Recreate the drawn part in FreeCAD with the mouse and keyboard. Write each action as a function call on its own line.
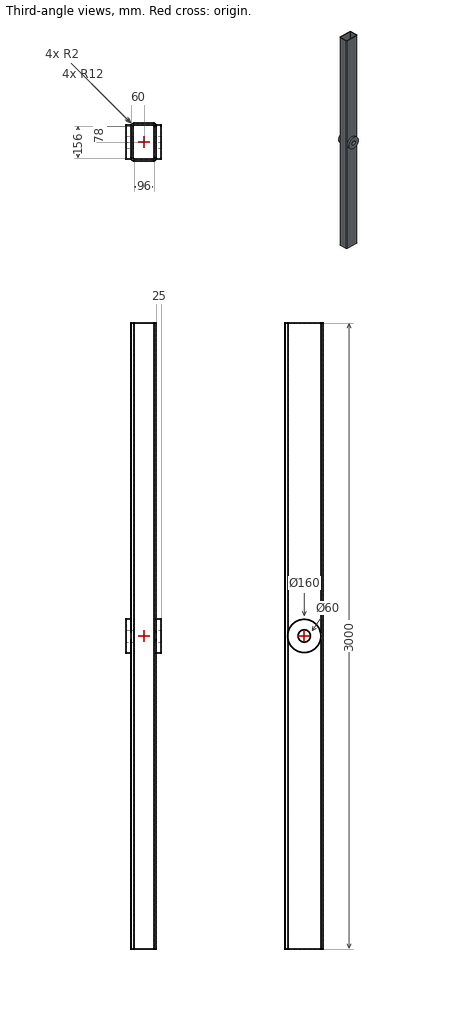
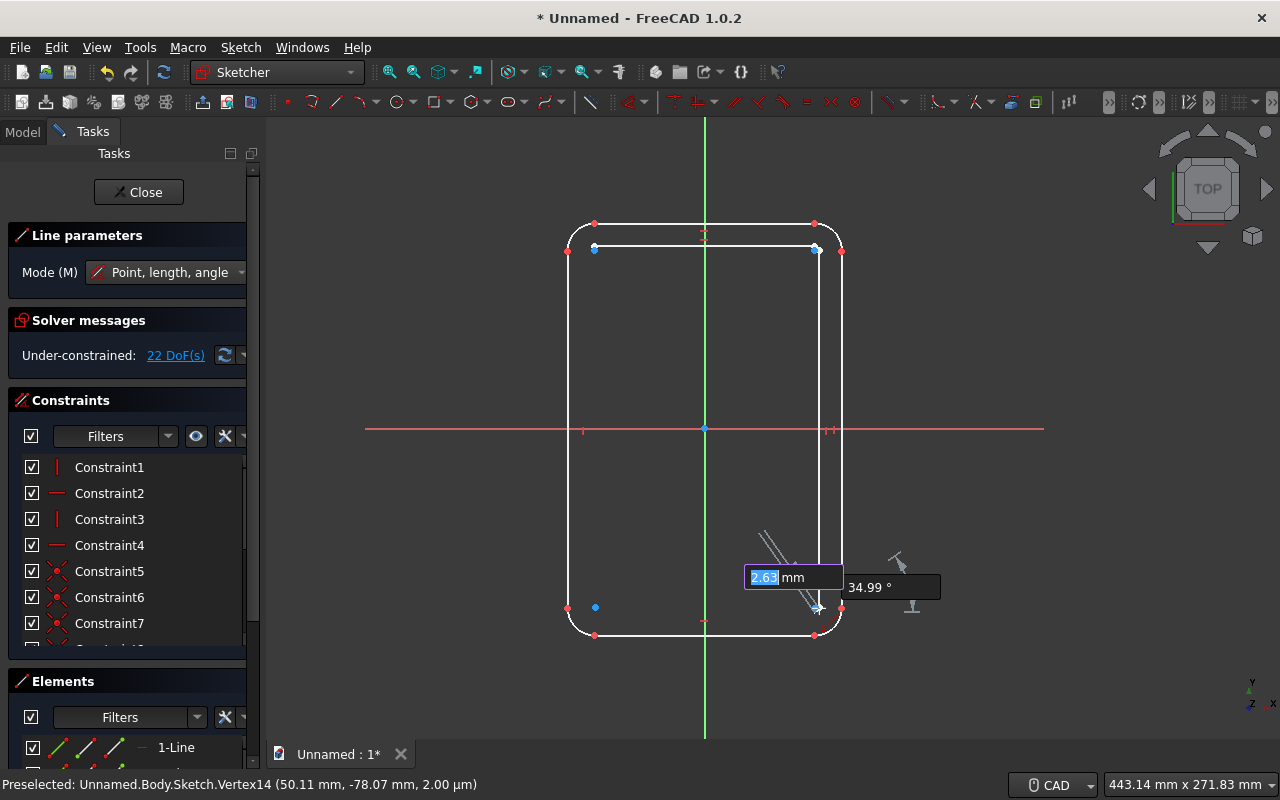
scroll(595, 612, up, 7)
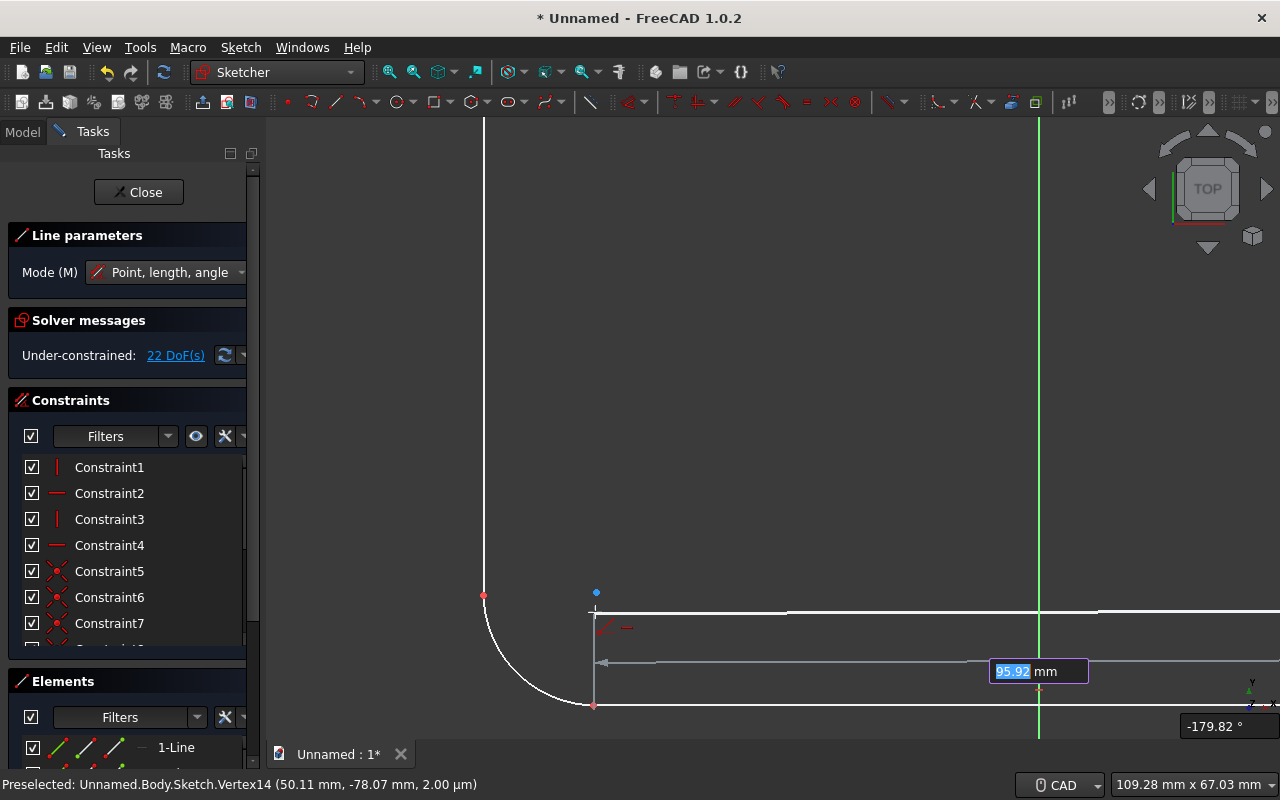
click(594, 610)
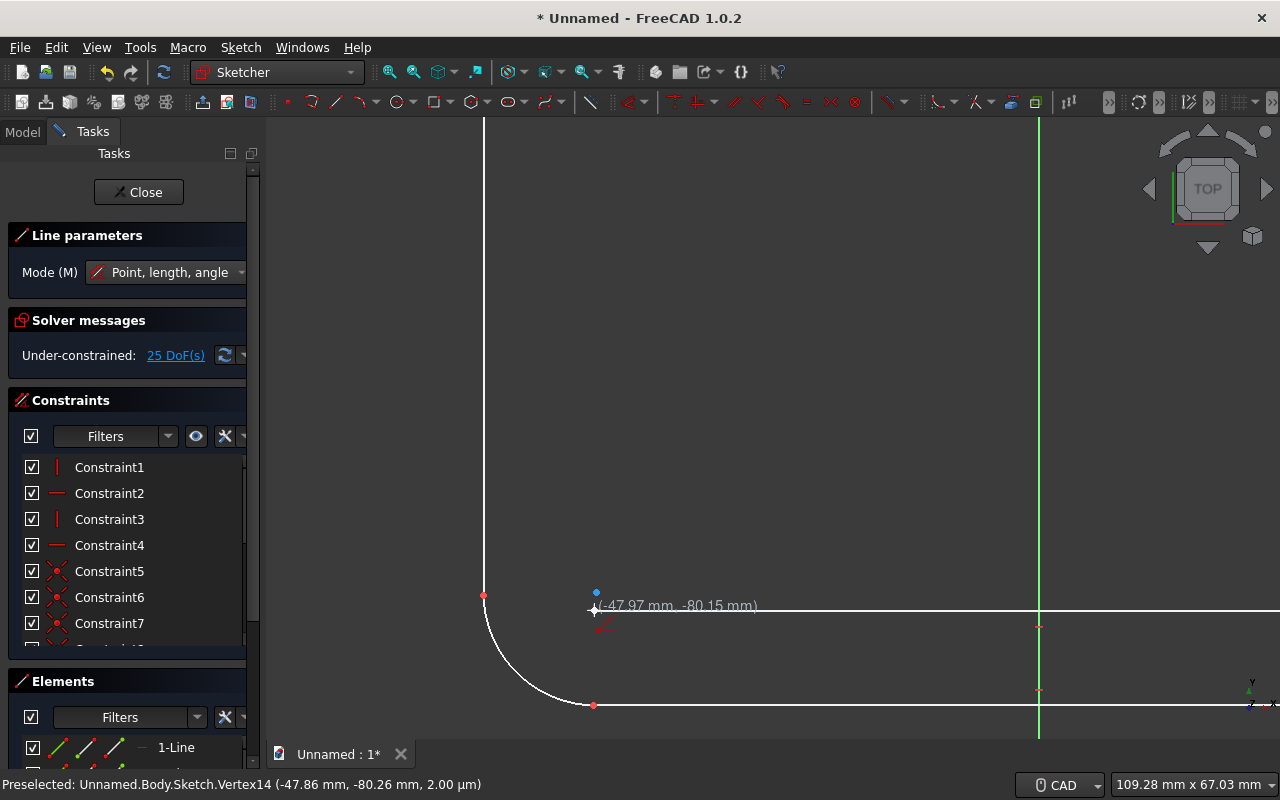
click(575, 591)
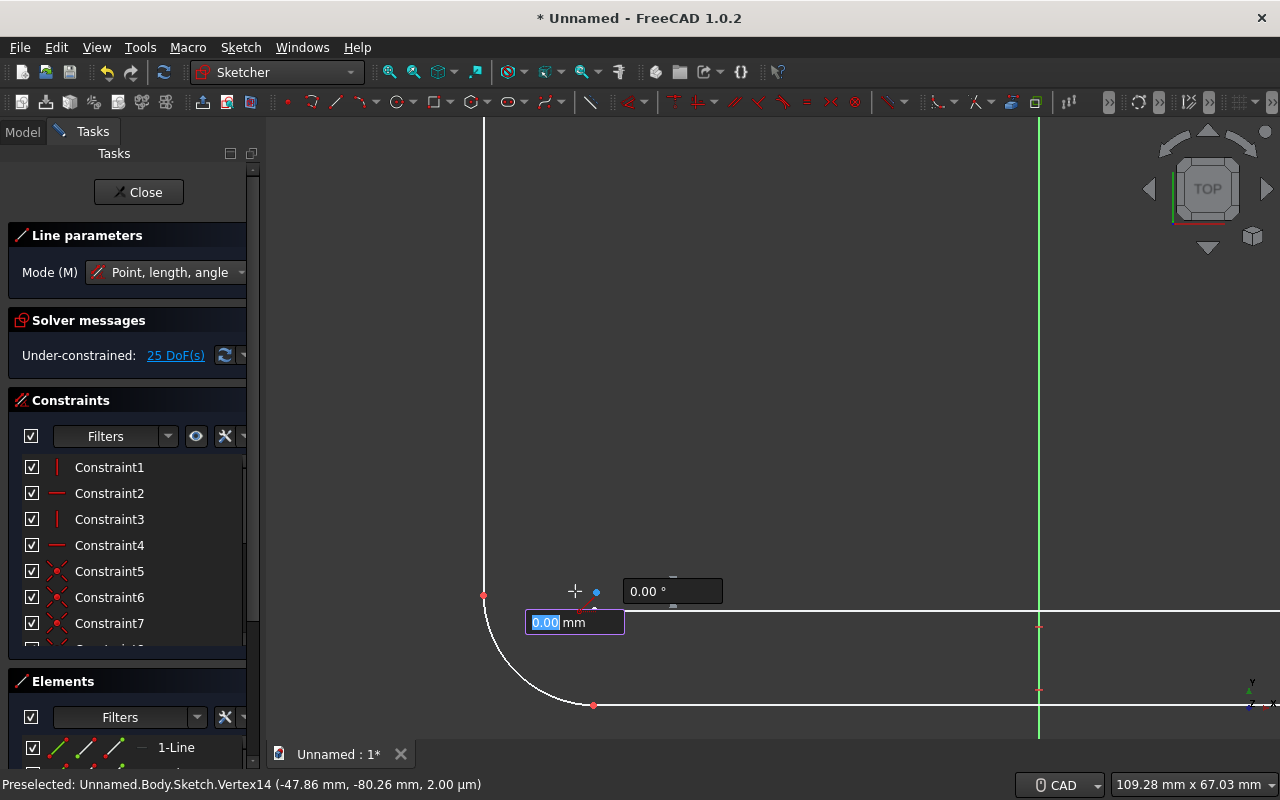
scroll(595, 612, down, 7)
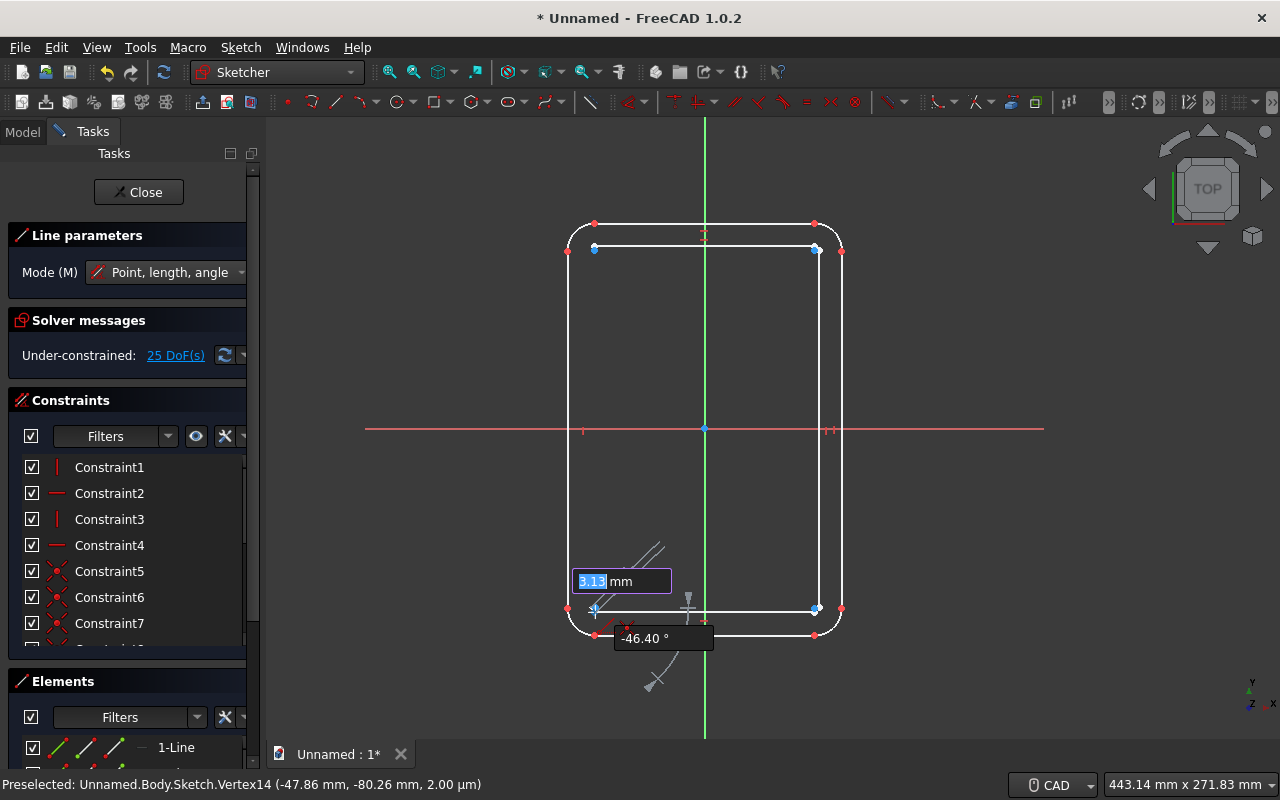
scroll(590, 250, up, 7)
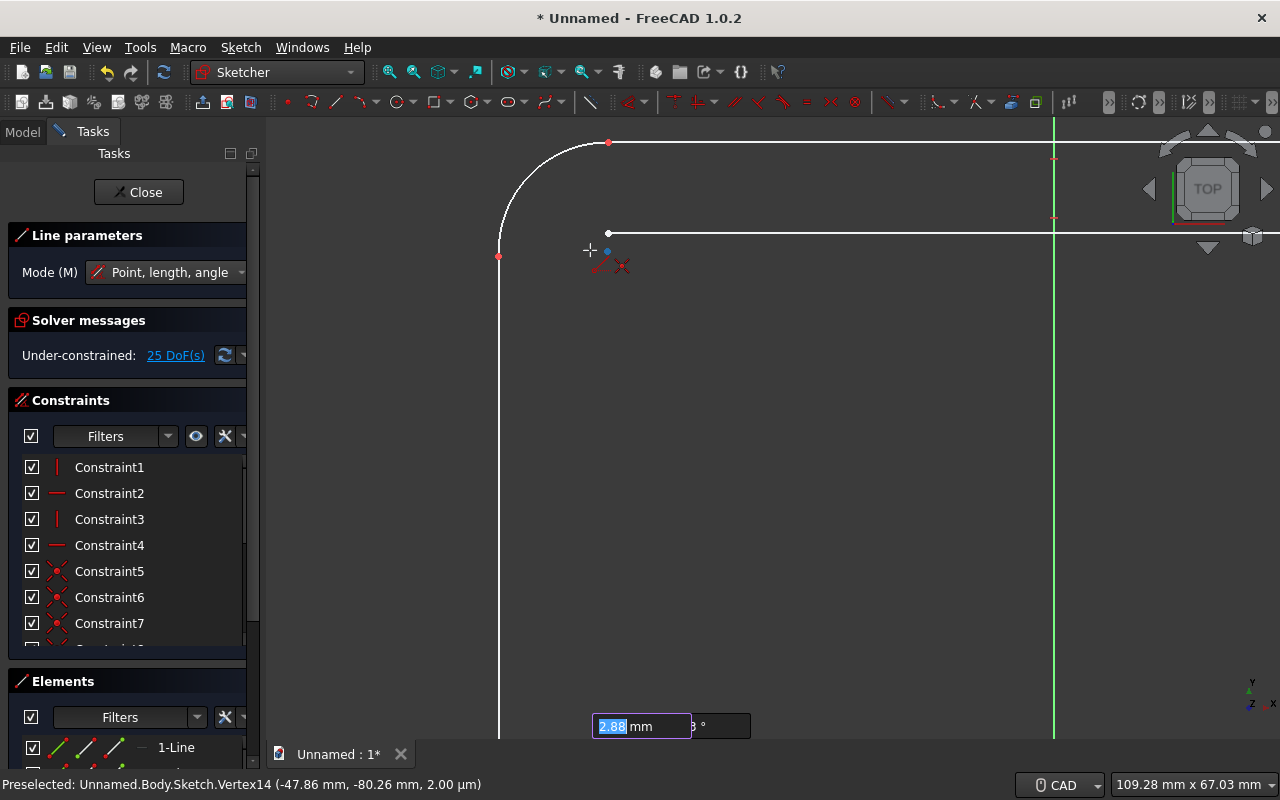
click(590, 251)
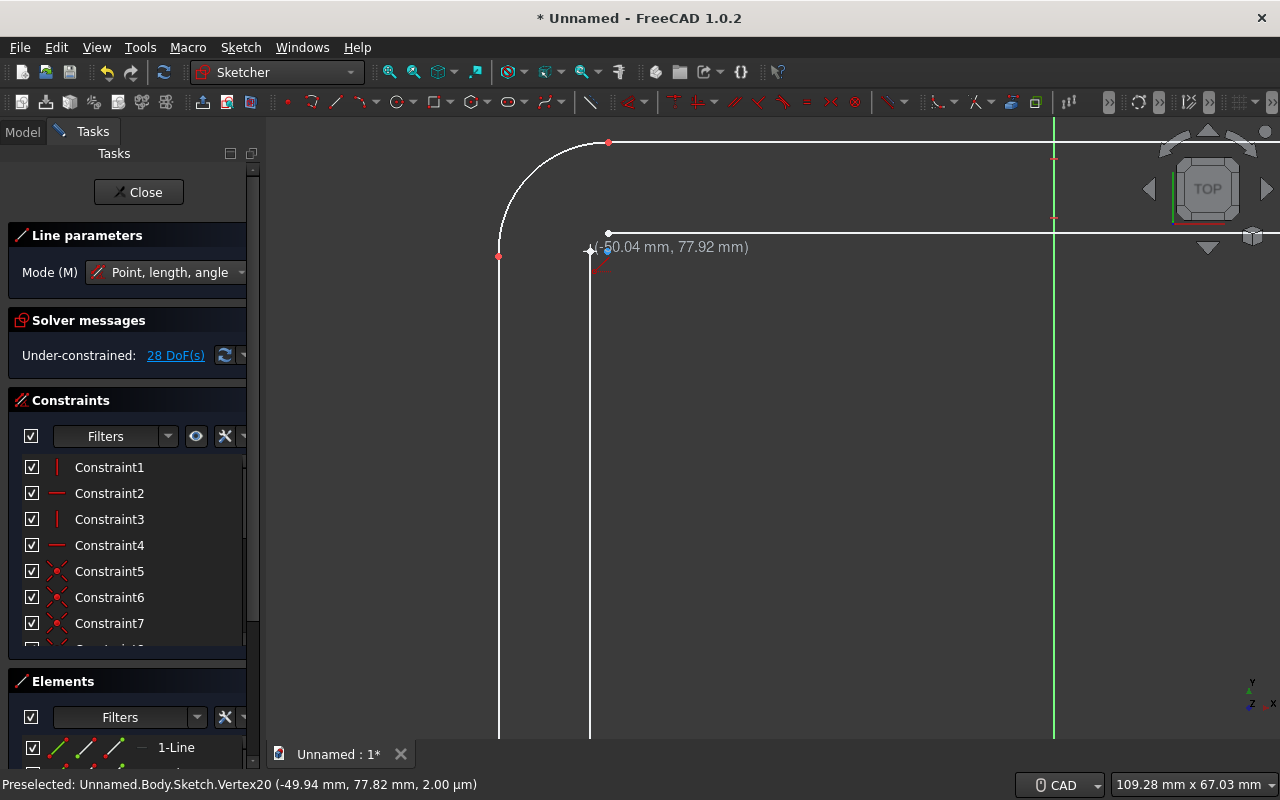
click(360, 102)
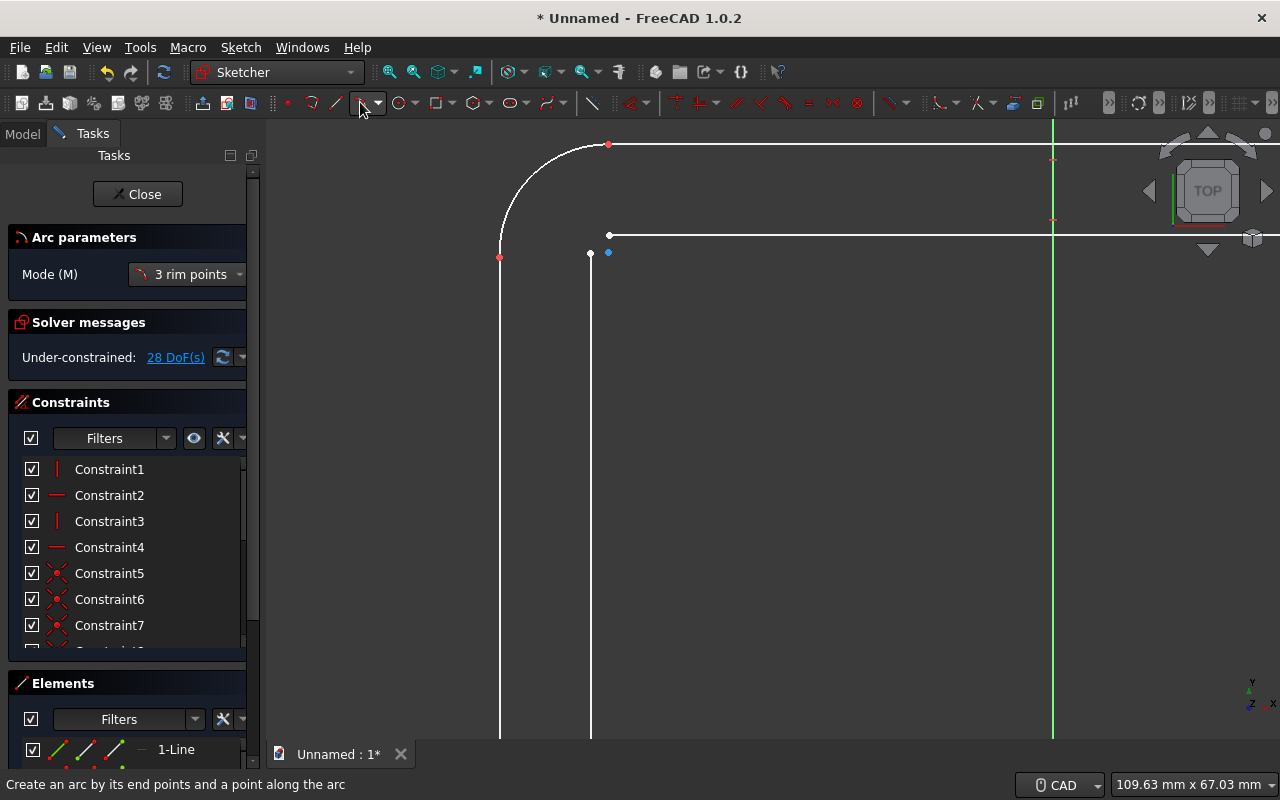
scroll(590, 251, down, 7)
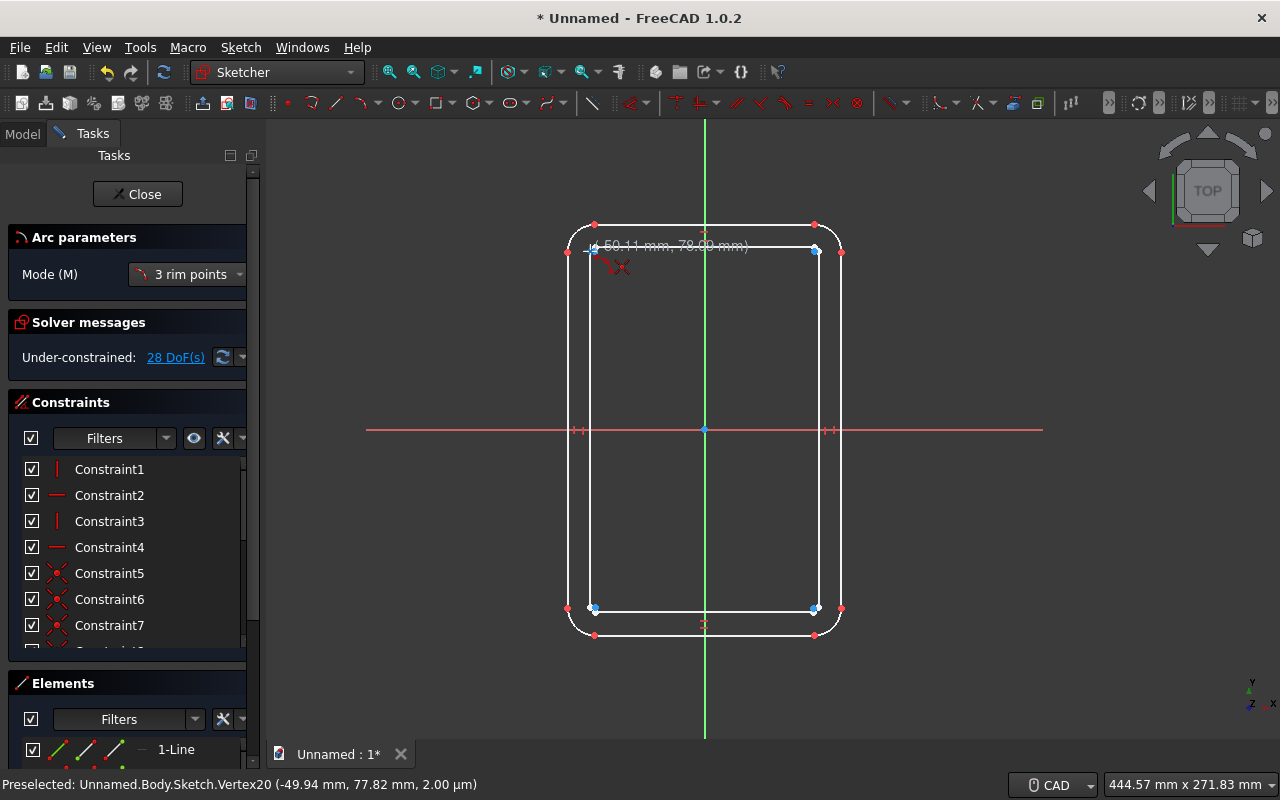
scroll(814, 247, up, 7)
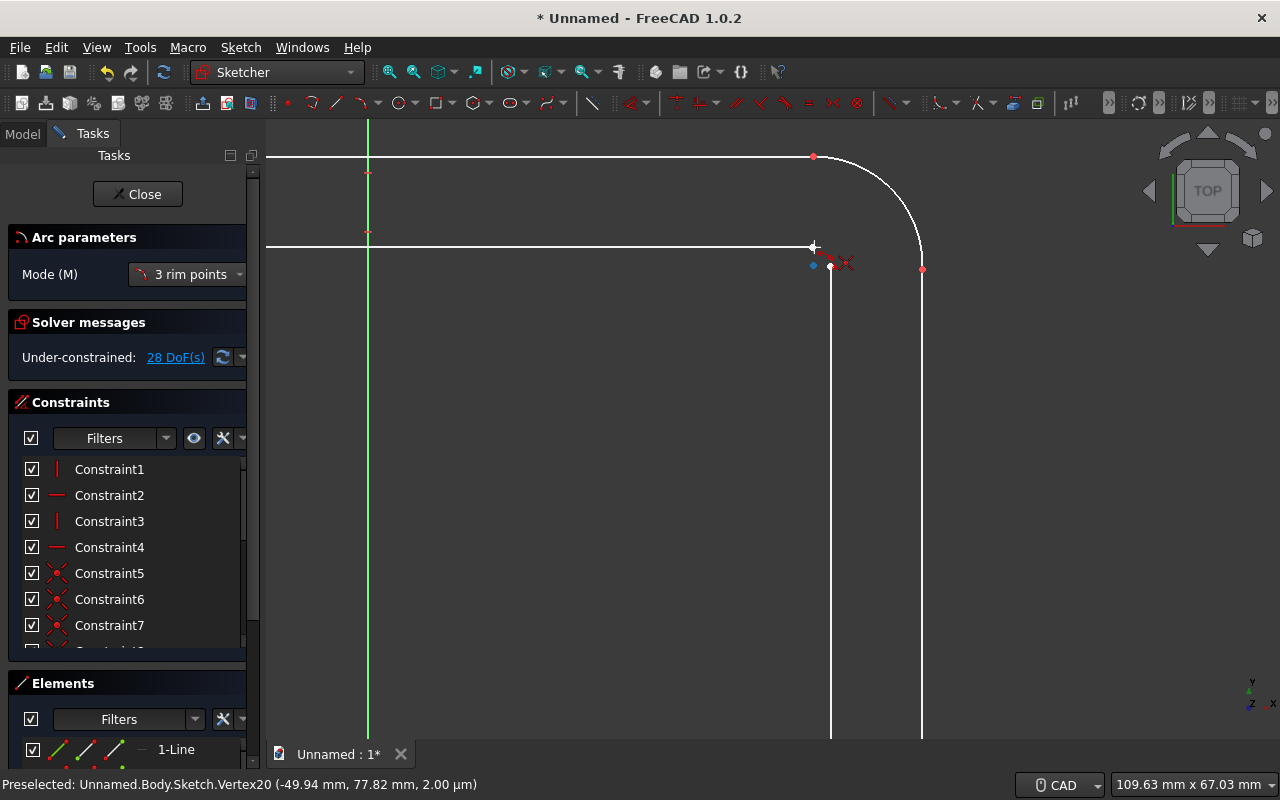
click(813, 247)
click(831, 267)